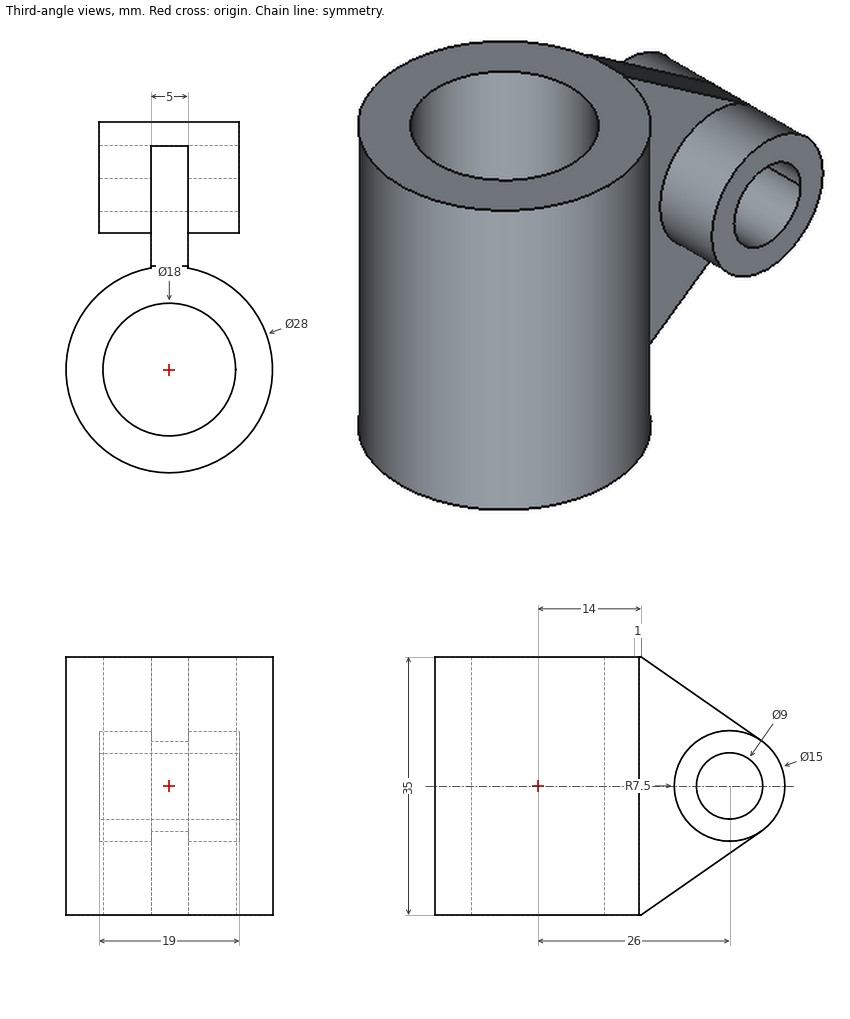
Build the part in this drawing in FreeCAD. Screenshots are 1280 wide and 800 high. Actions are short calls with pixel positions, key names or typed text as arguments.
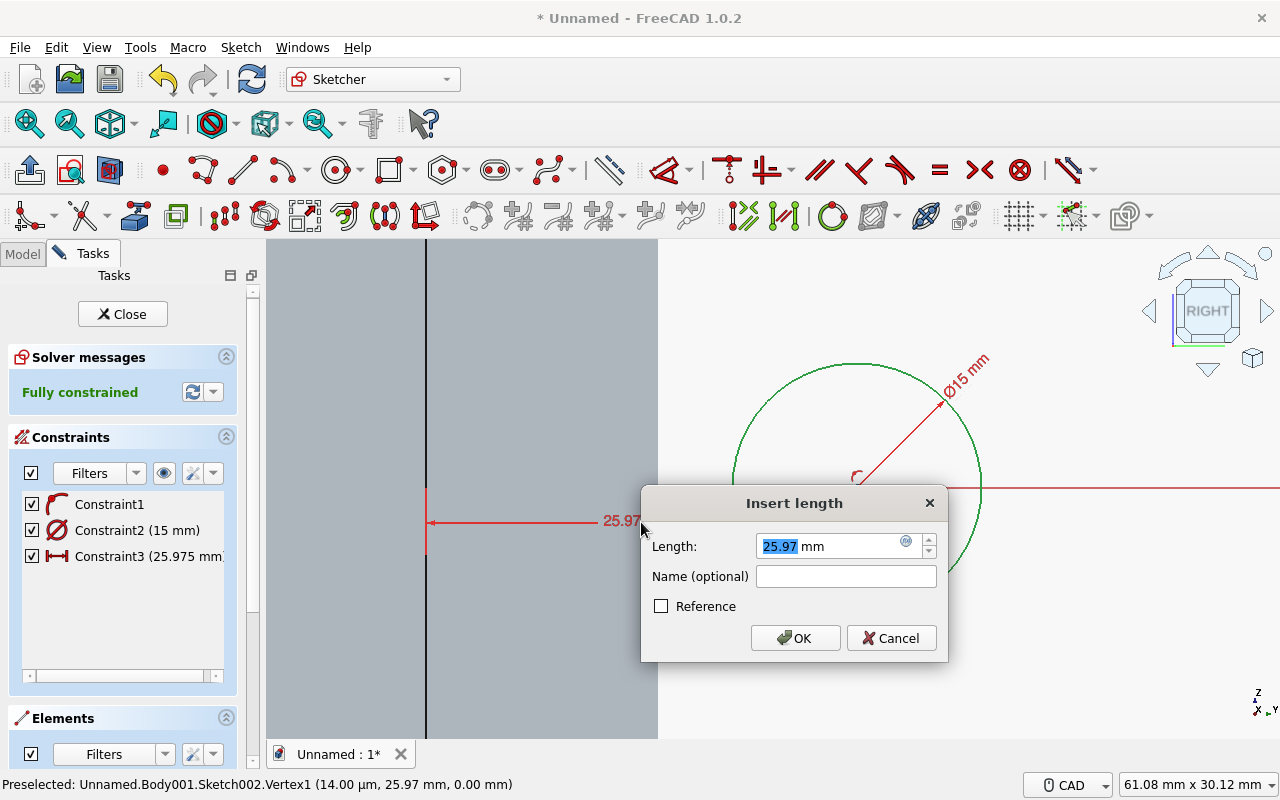
text(26)
key(Return)
key(Escape)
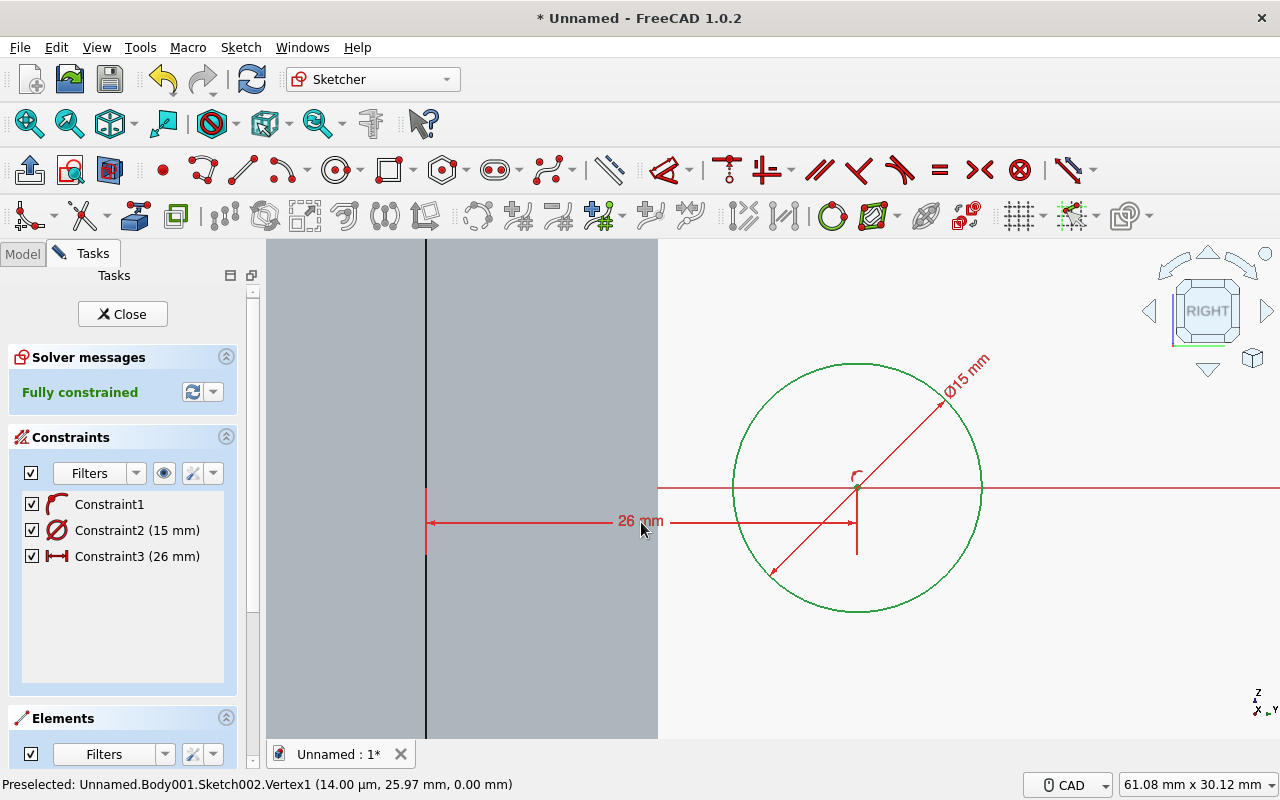
click(123, 314)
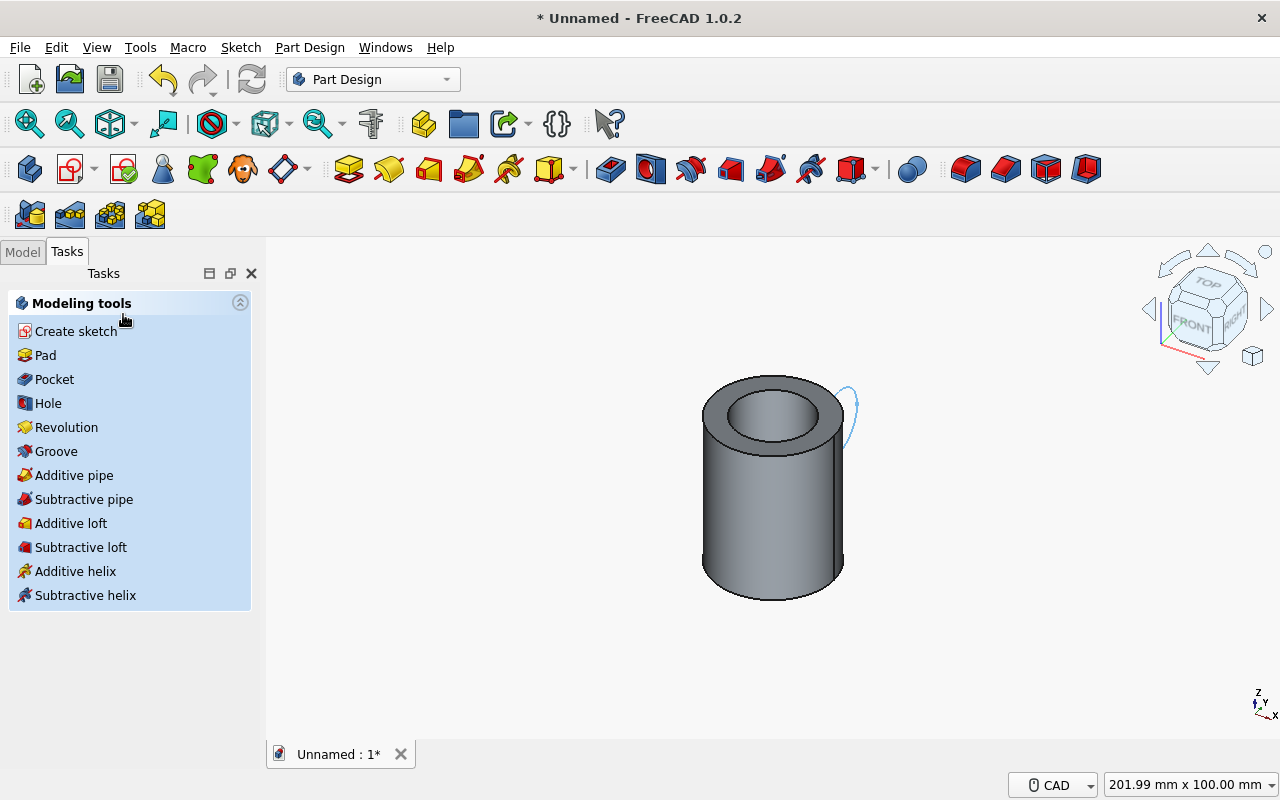
click(350, 170)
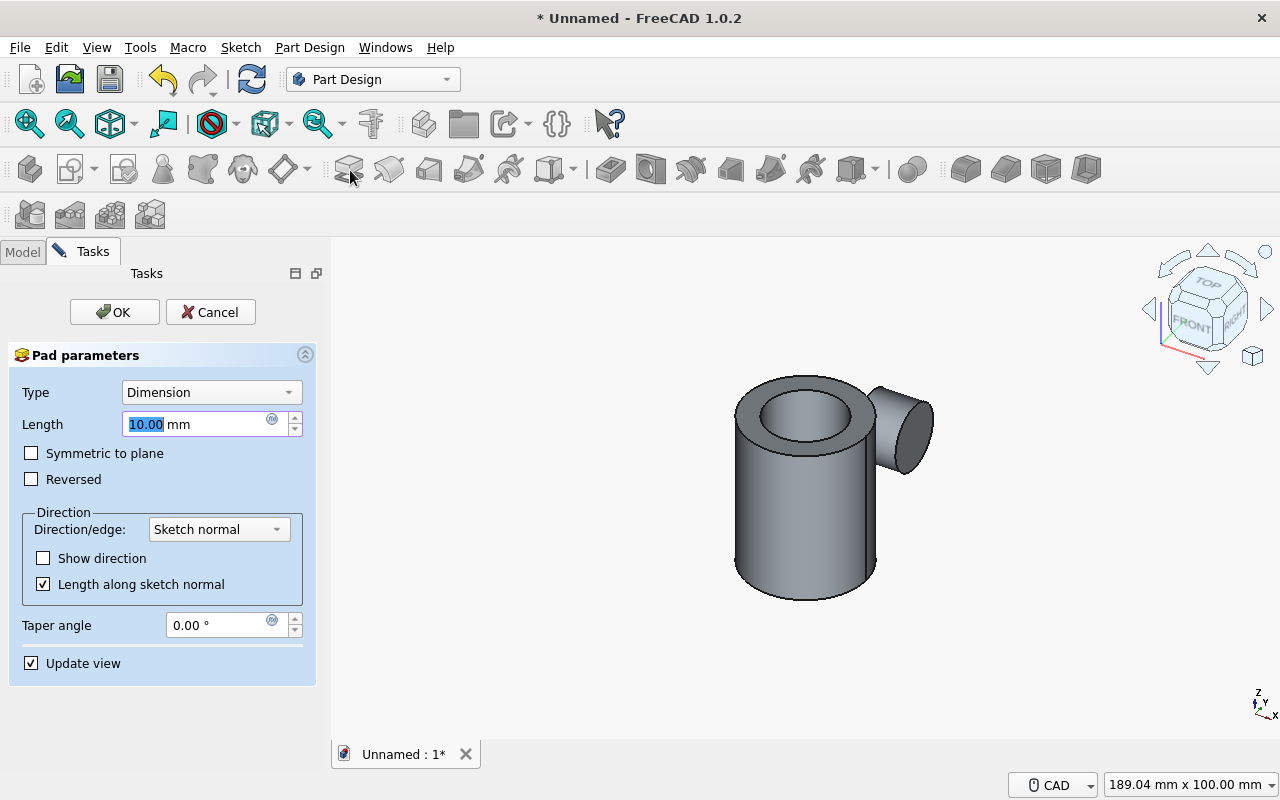
text(19)
key(Tab)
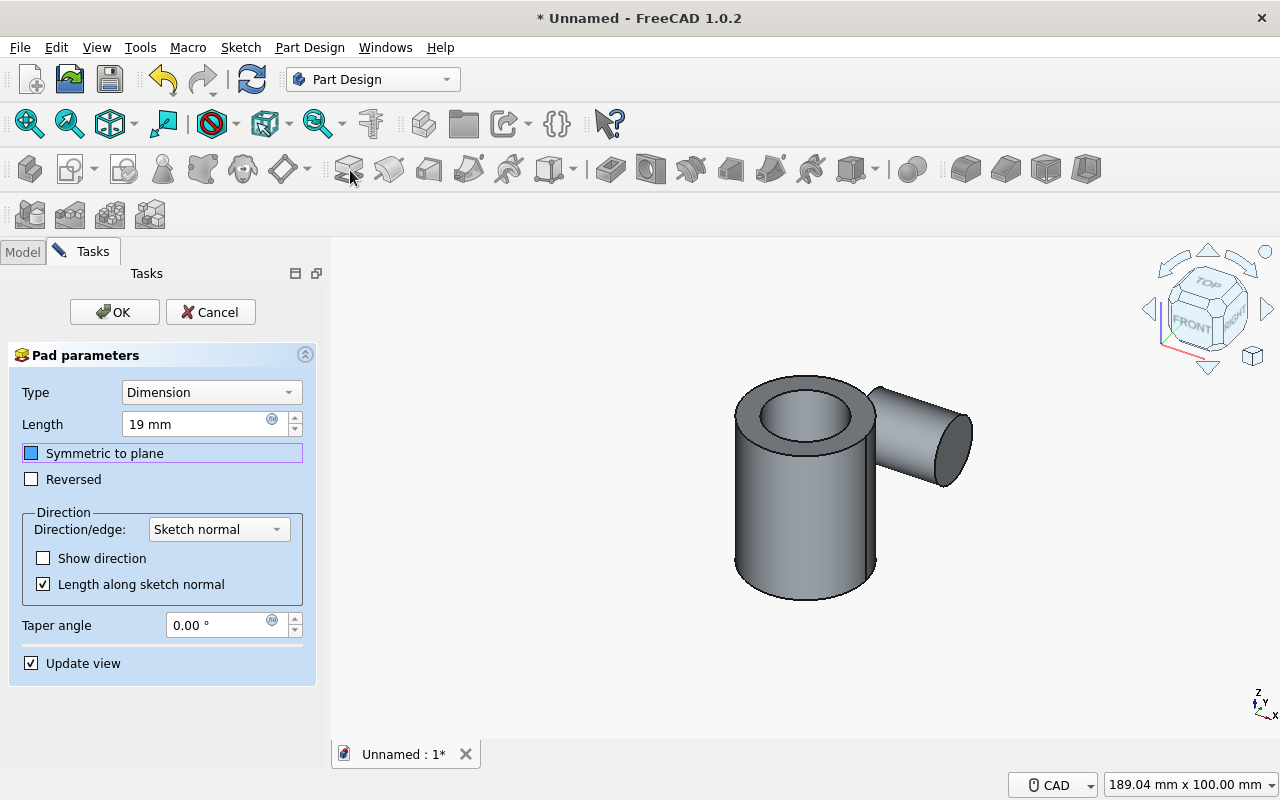
click(30, 453)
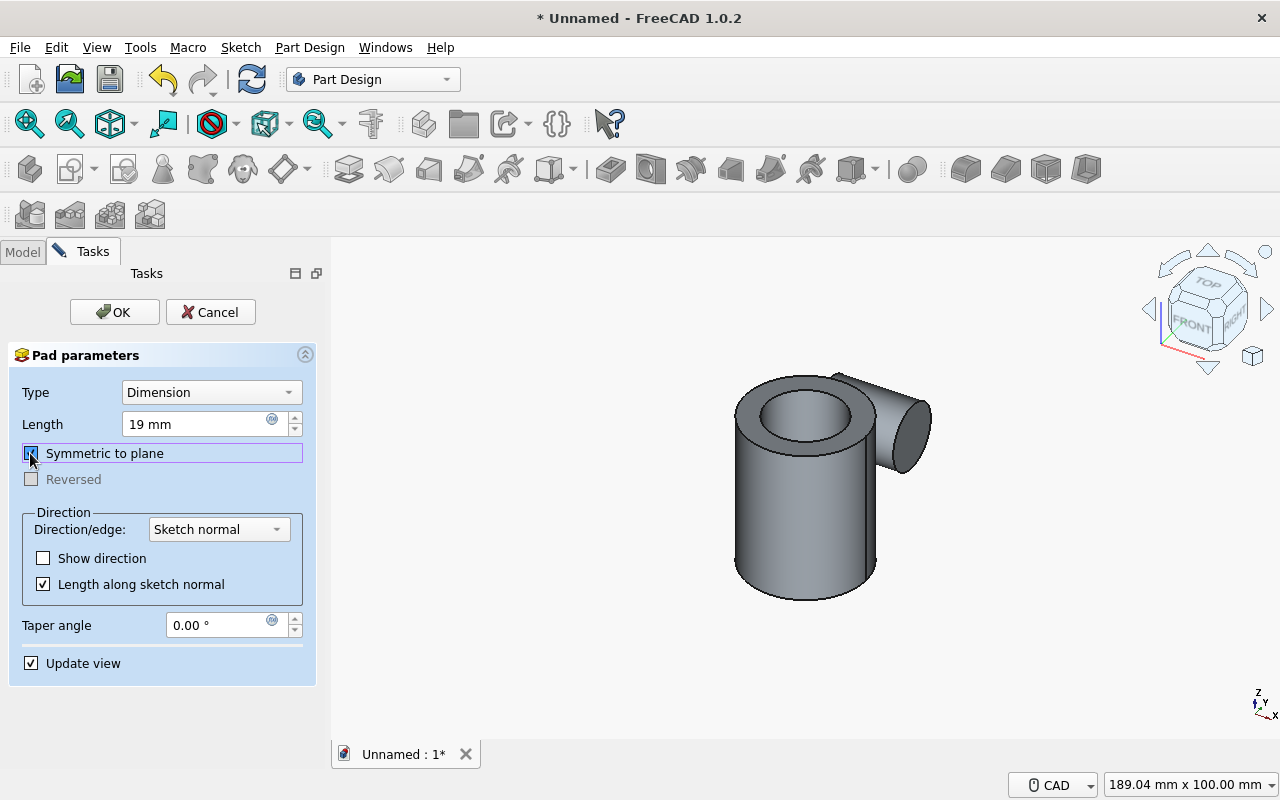
click(115, 312)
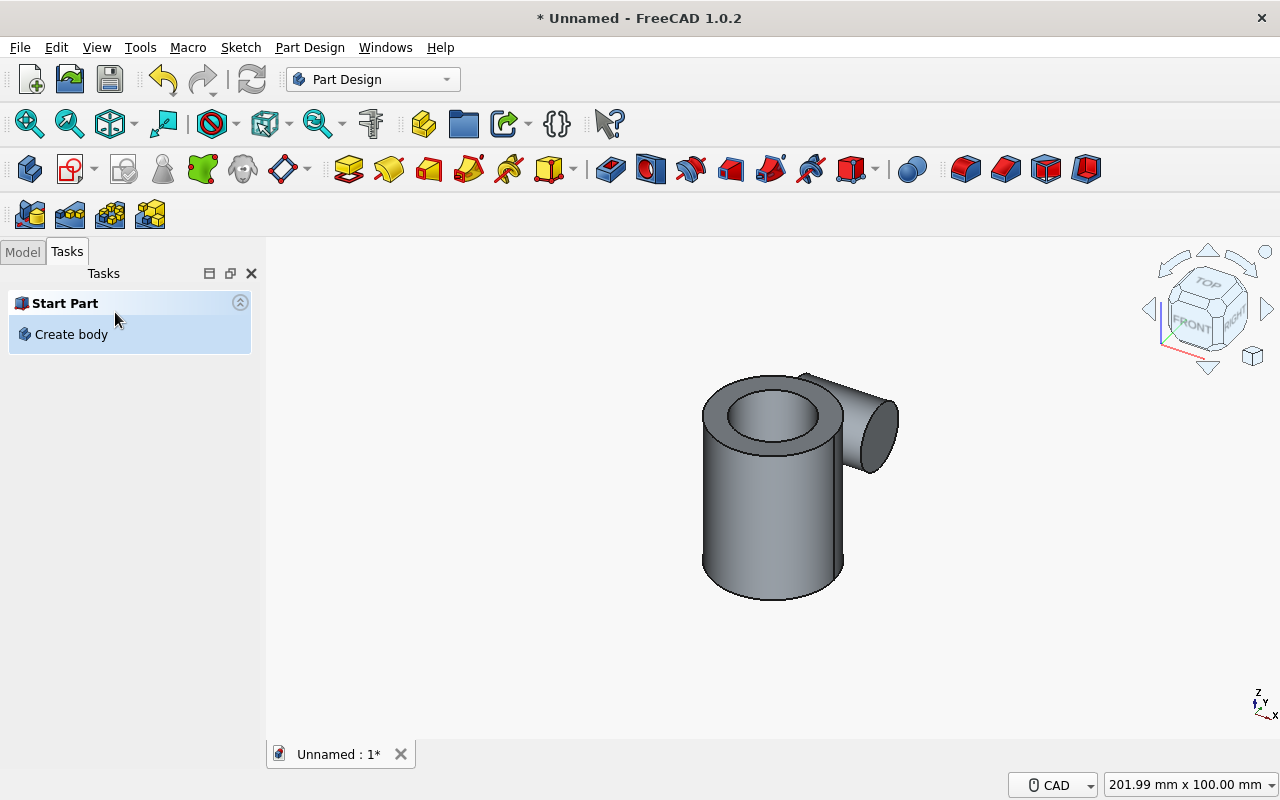
key(v)
key(f)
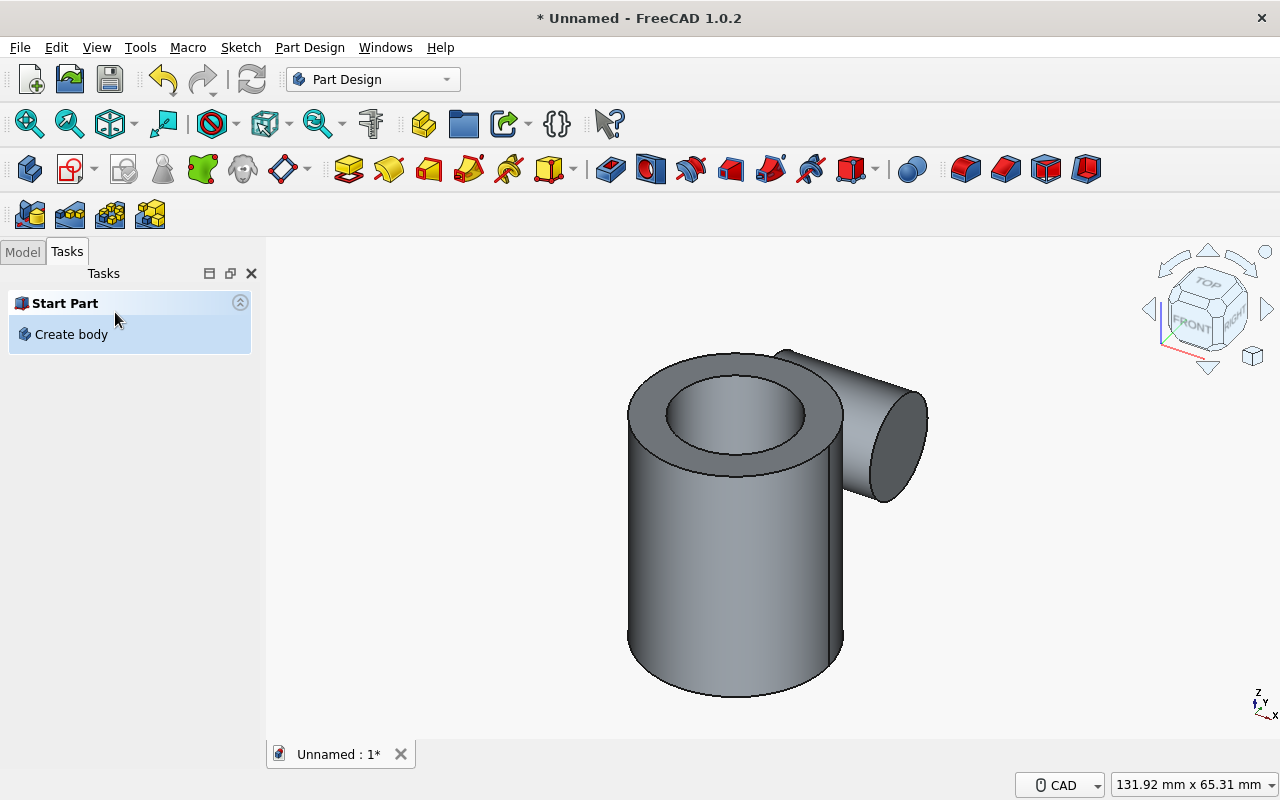
click(899, 446)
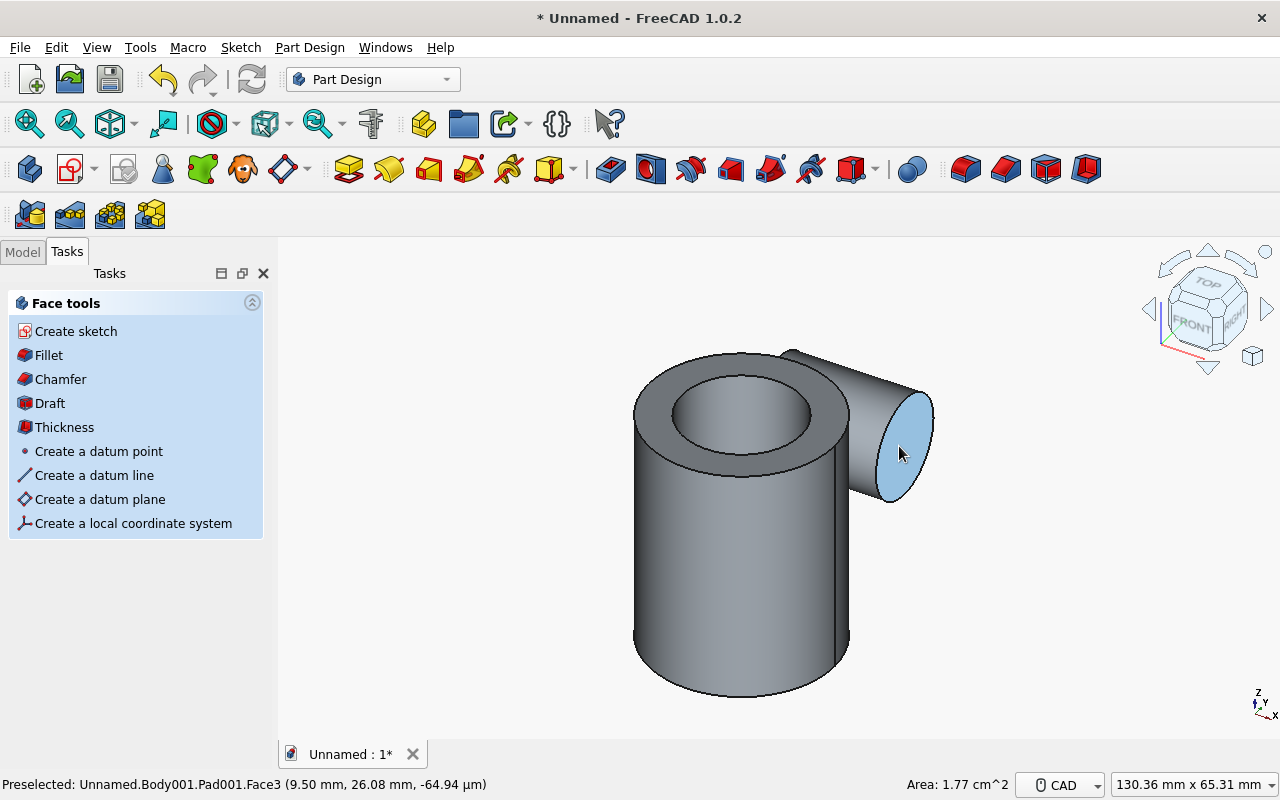
click(70, 170)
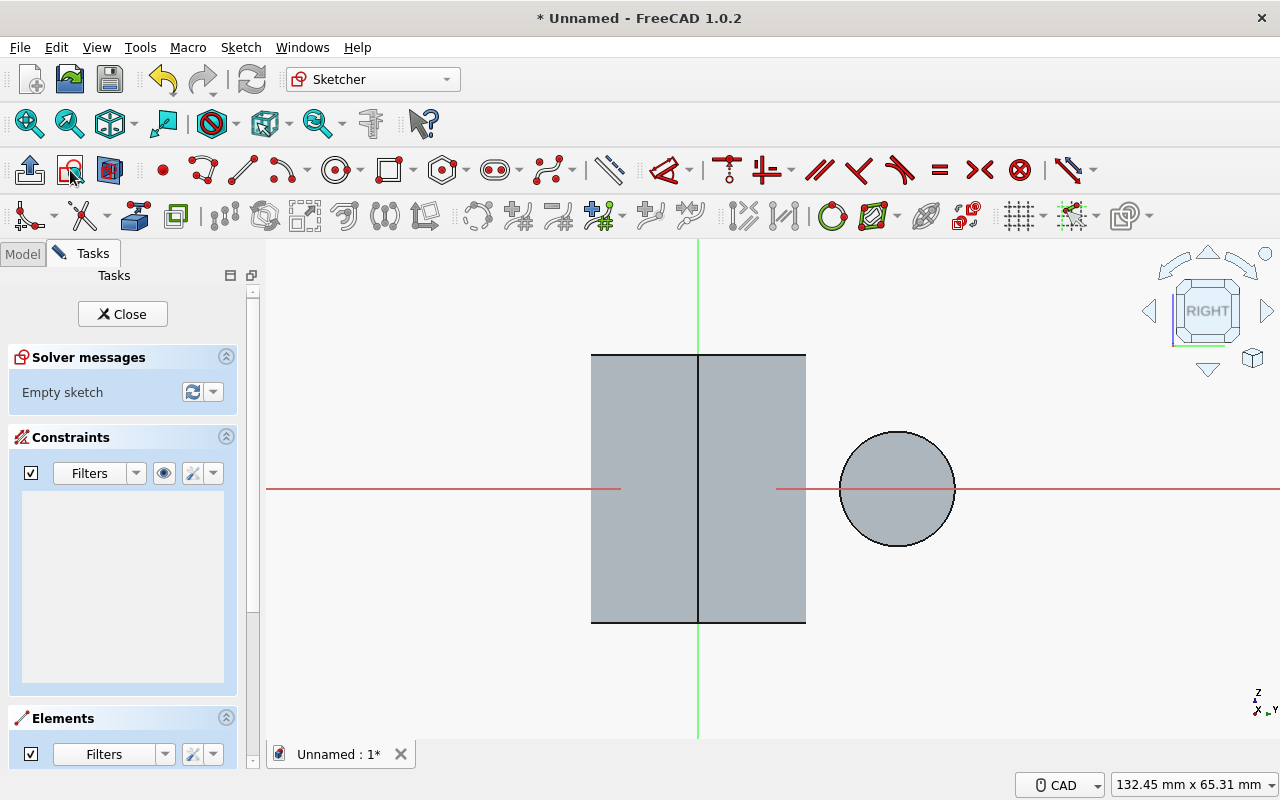
scroll(946, 489, up, 8)